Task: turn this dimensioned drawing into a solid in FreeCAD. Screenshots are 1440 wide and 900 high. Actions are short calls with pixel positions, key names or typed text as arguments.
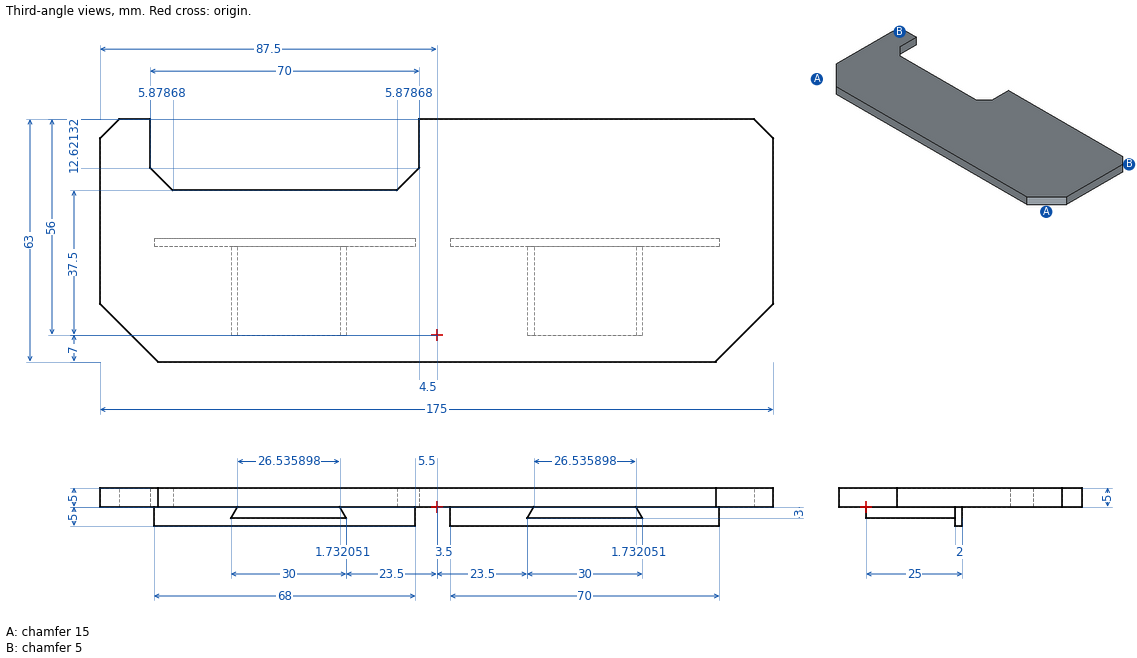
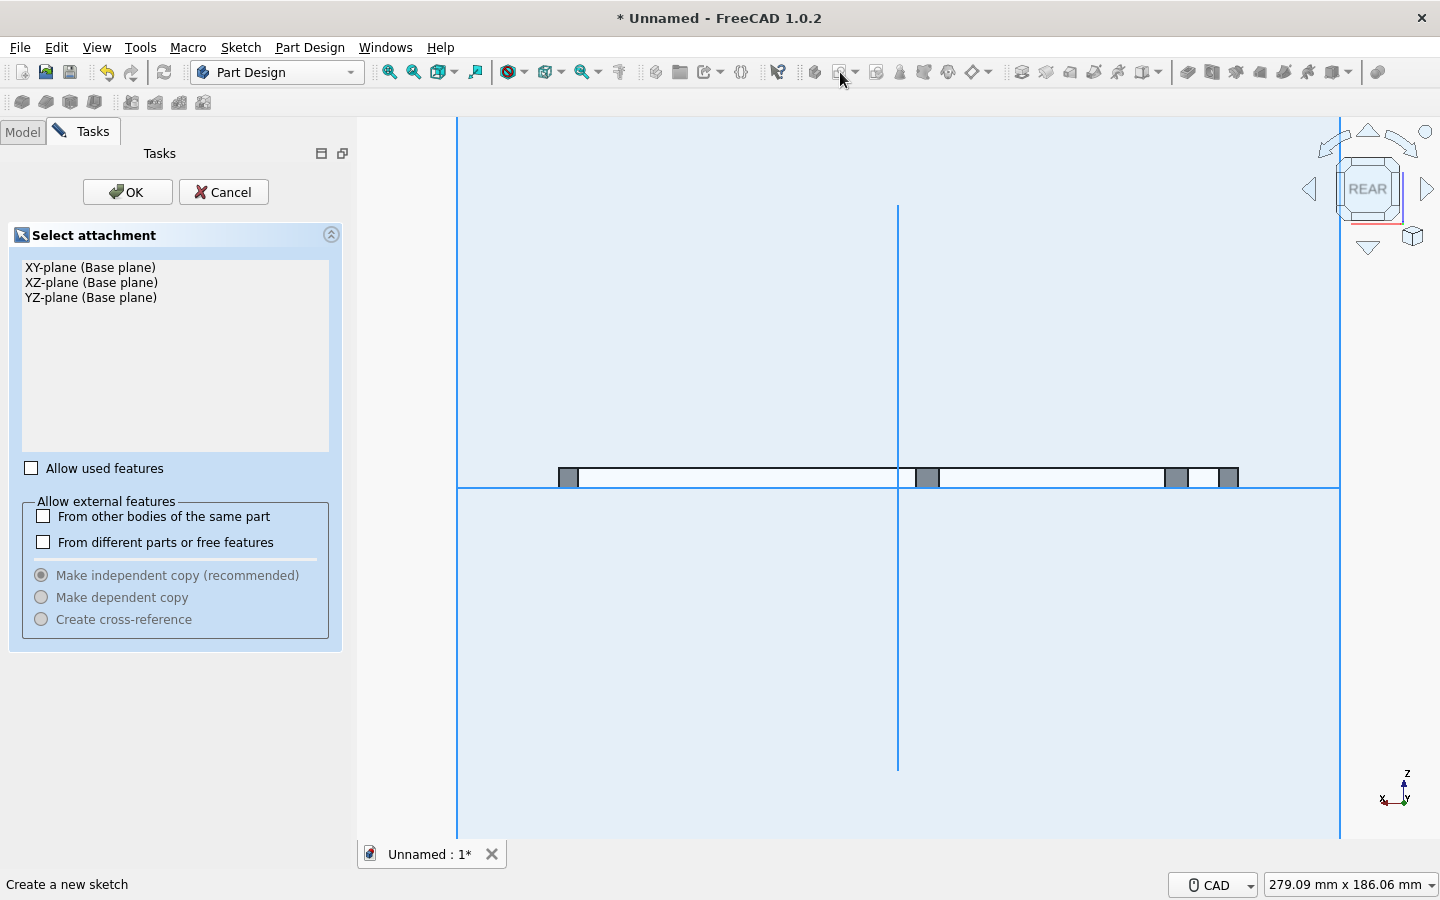
click(82, 282)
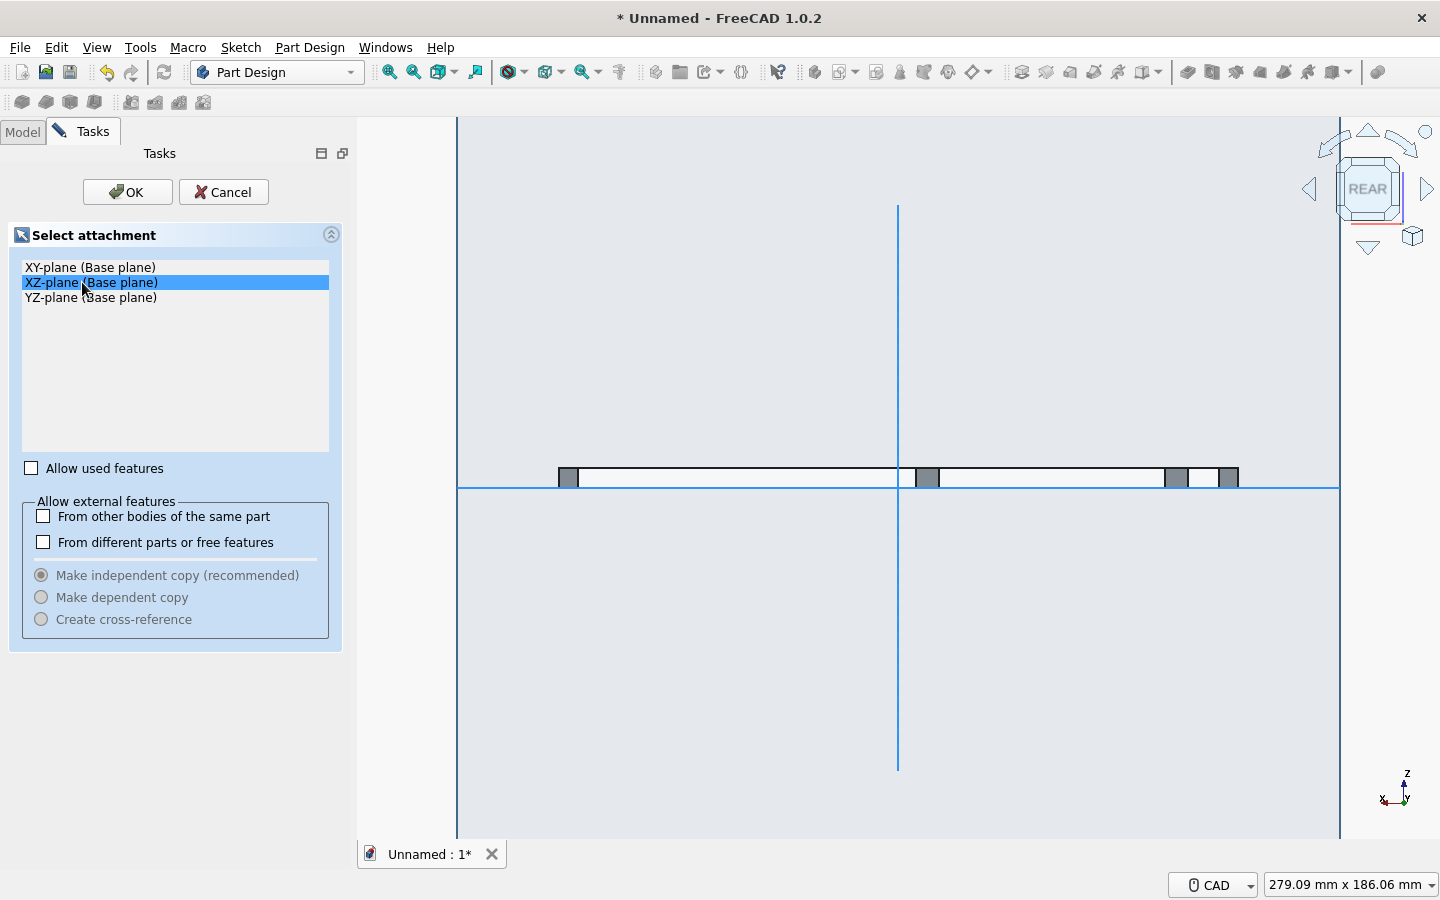
click(128, 192)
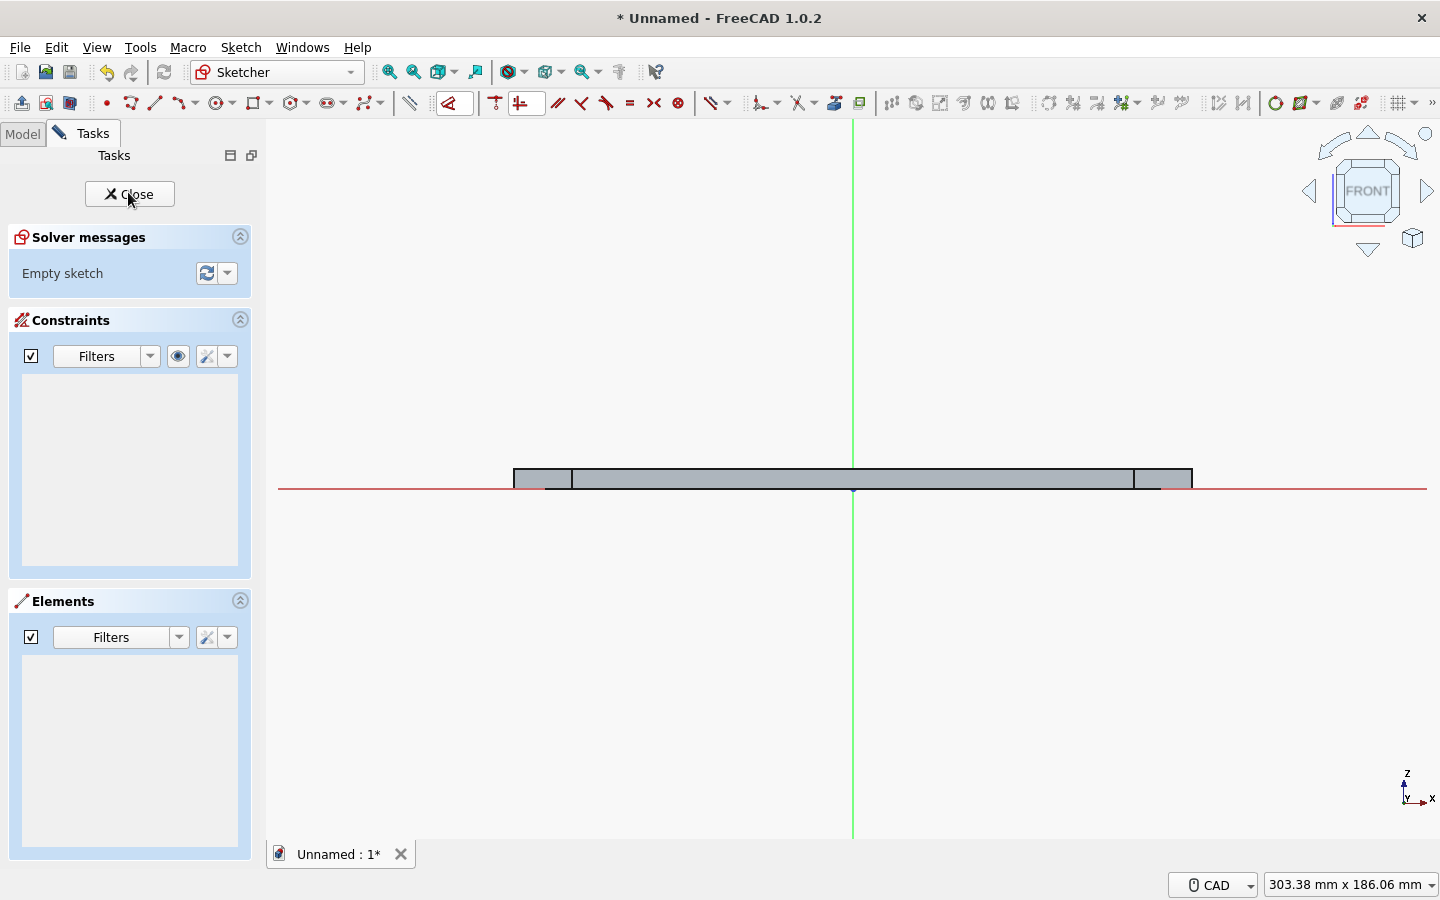
click(70, 104)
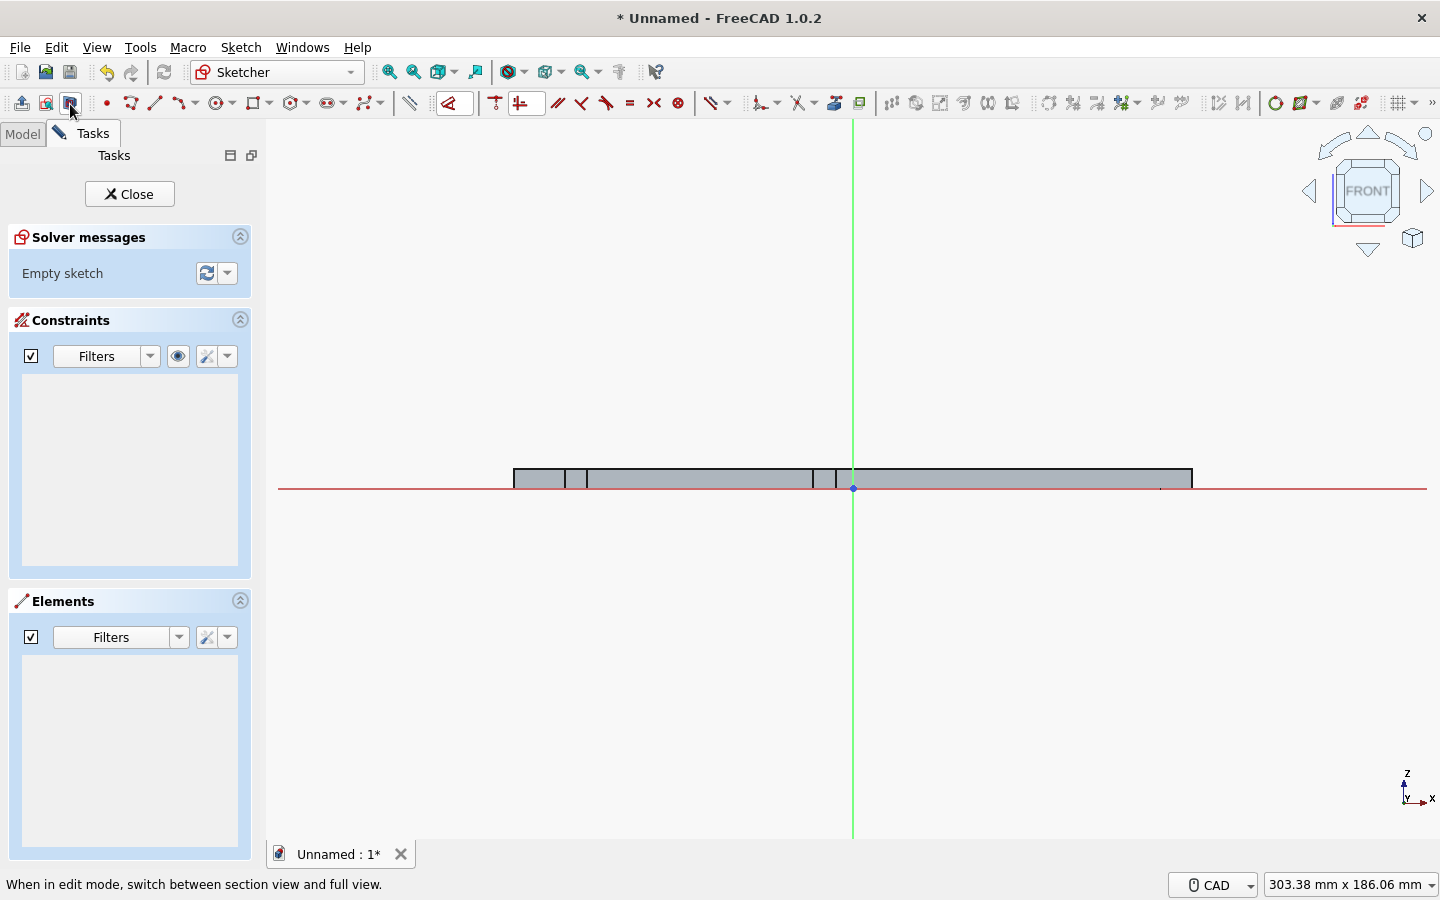
scroll(936, 513, up, 3)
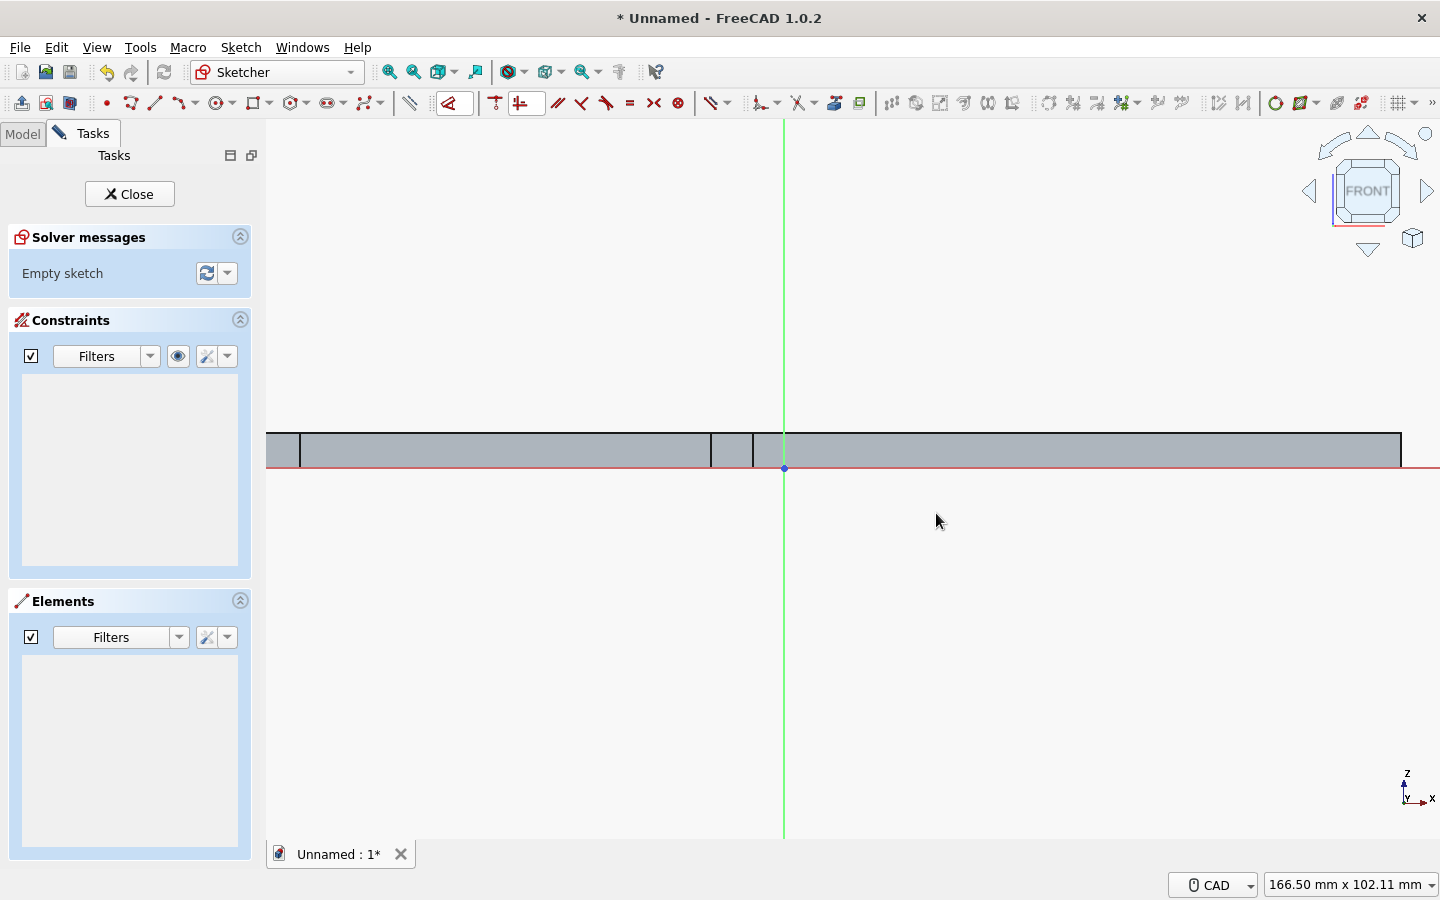
click(132, 104)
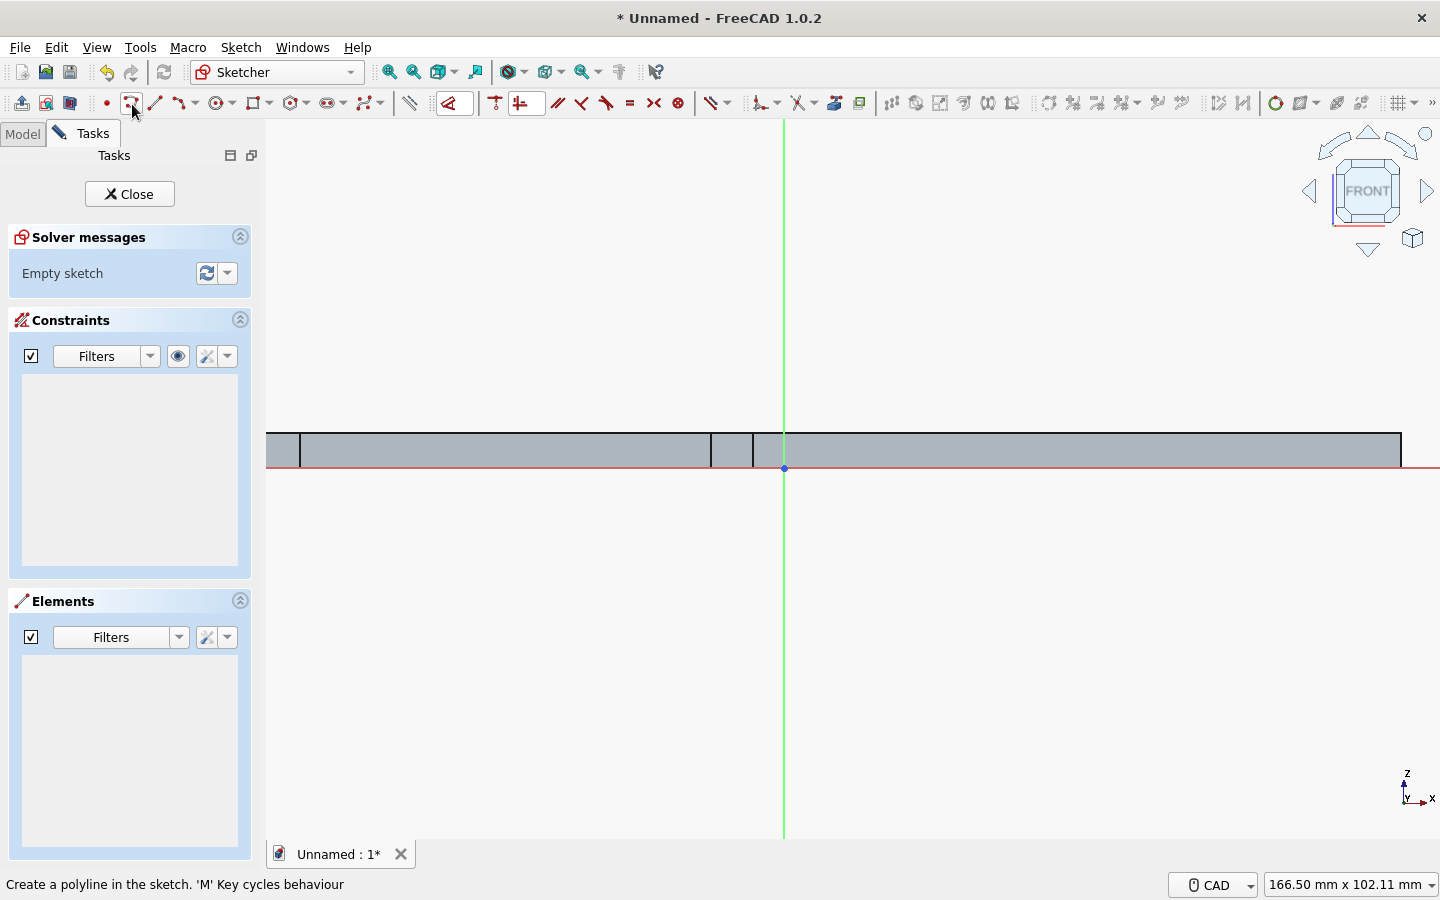
click(950, 489)
click(1162, 489)
click(1149, 468)
click(962, 477)
click(950, 490)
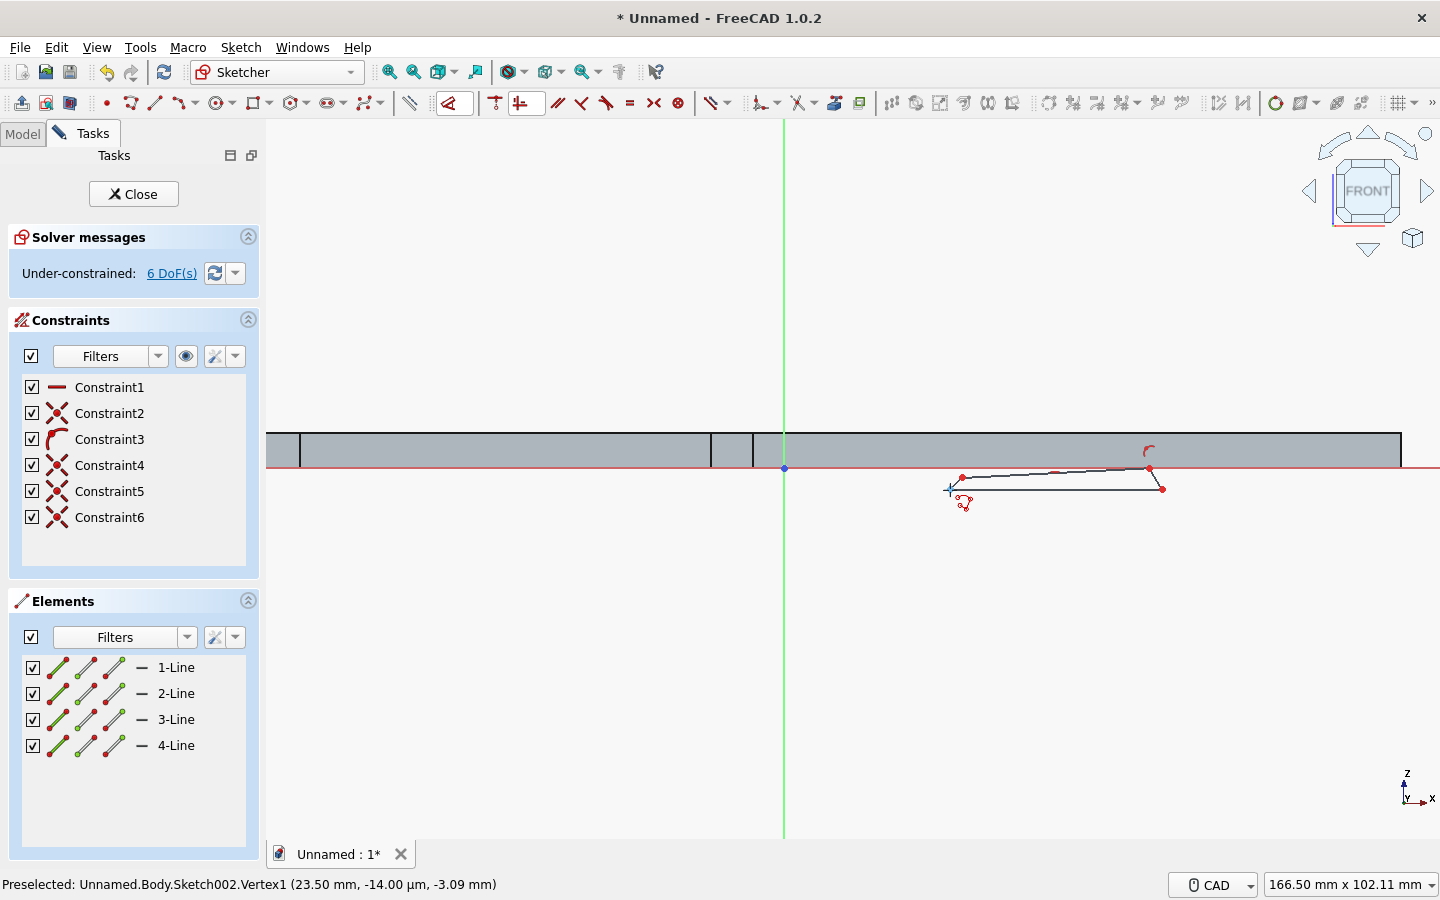
click(619, 489)
click(606, 468)
click(419, 477)
click(407, 489)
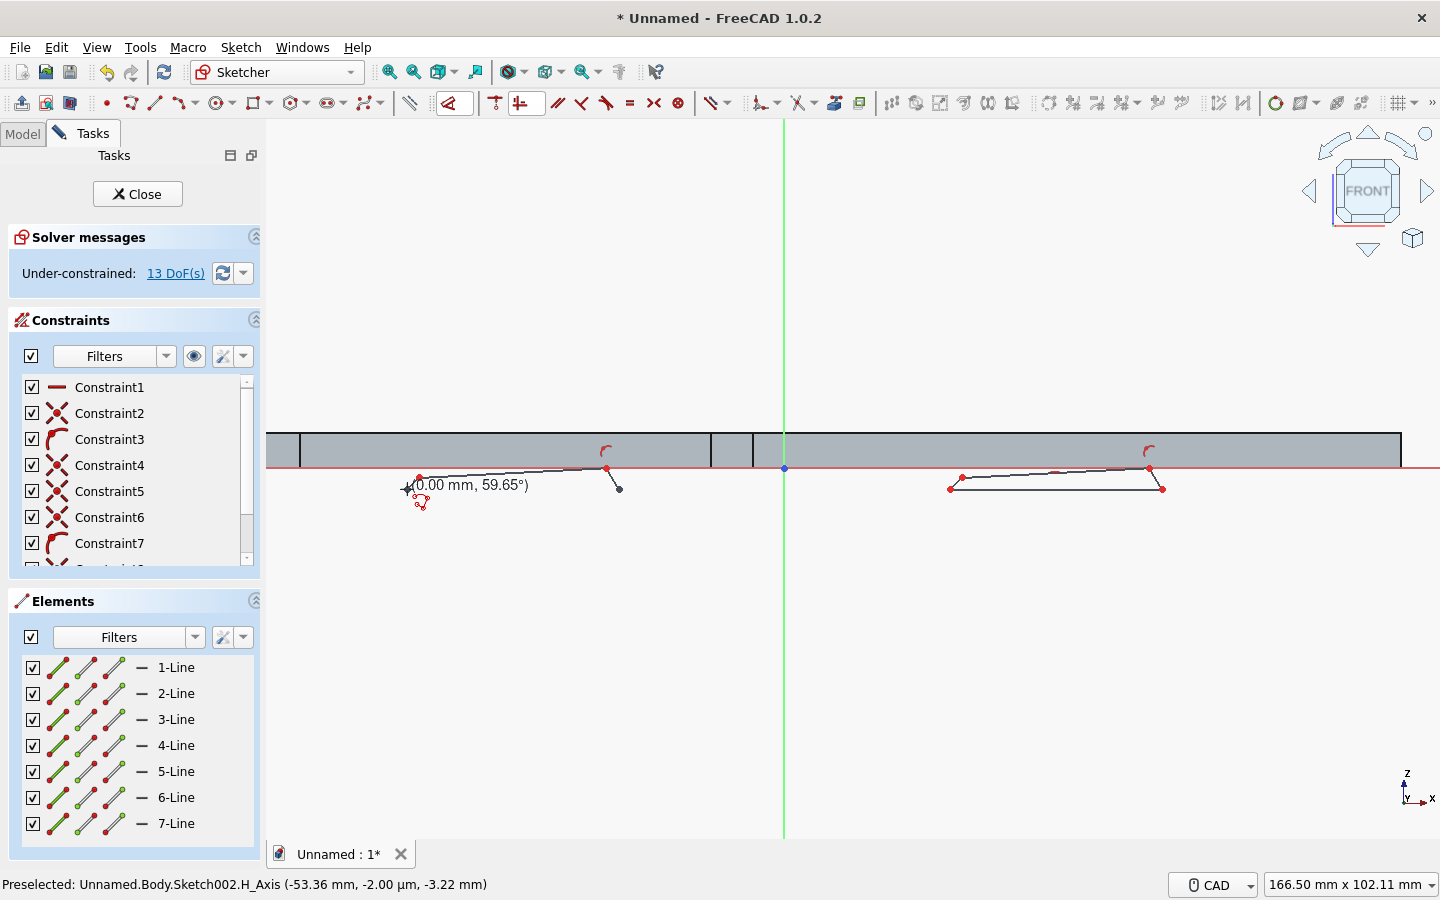
scroll(619, 489, up, 2)